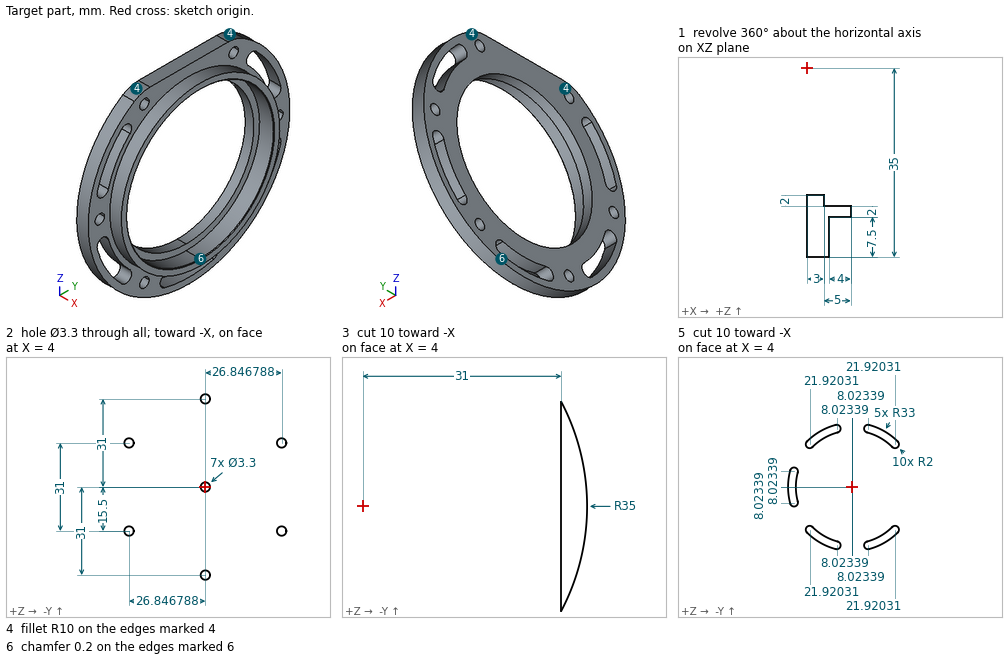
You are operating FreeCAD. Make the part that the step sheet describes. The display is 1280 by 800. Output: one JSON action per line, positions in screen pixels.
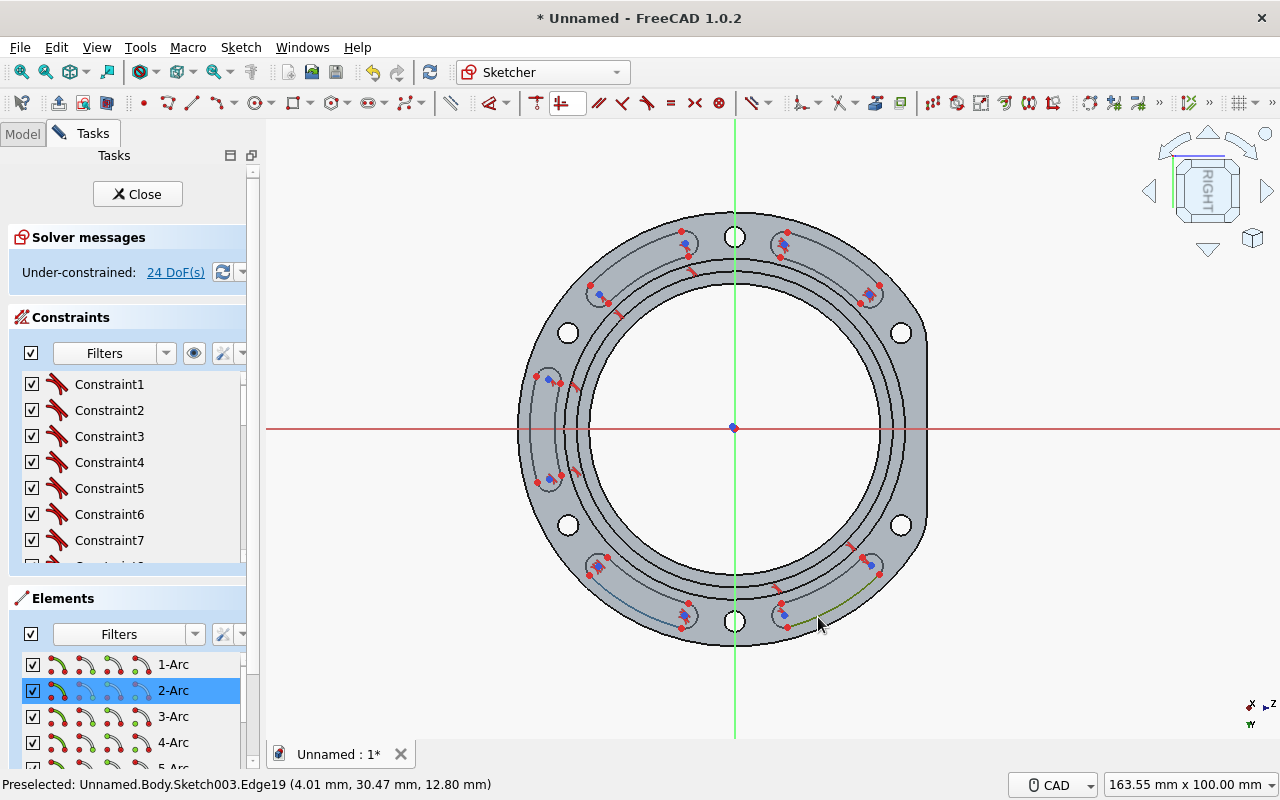
{"action": "left_click", "coordinate": [536, 104]}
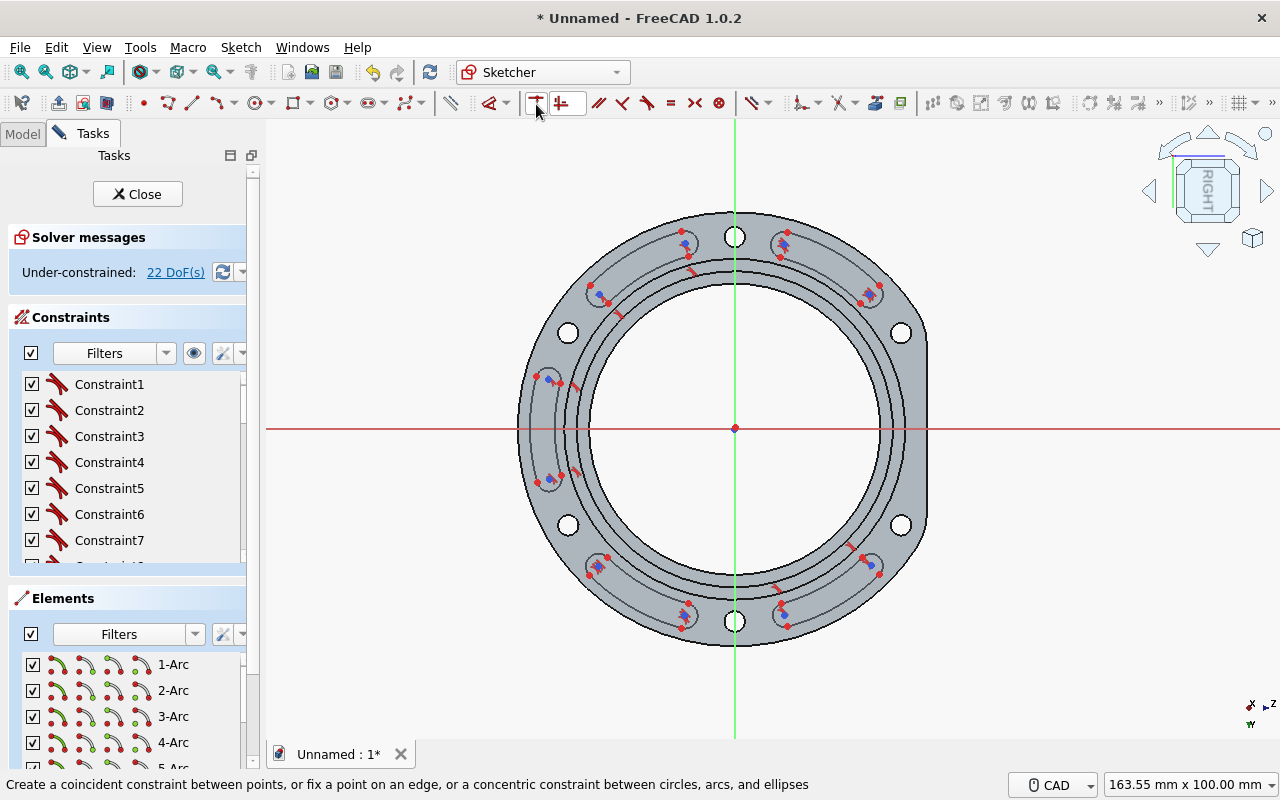
{"action": "scroll", "coordinate": [735, 429], "scroll_direction": "up", "scroll_amount": 7}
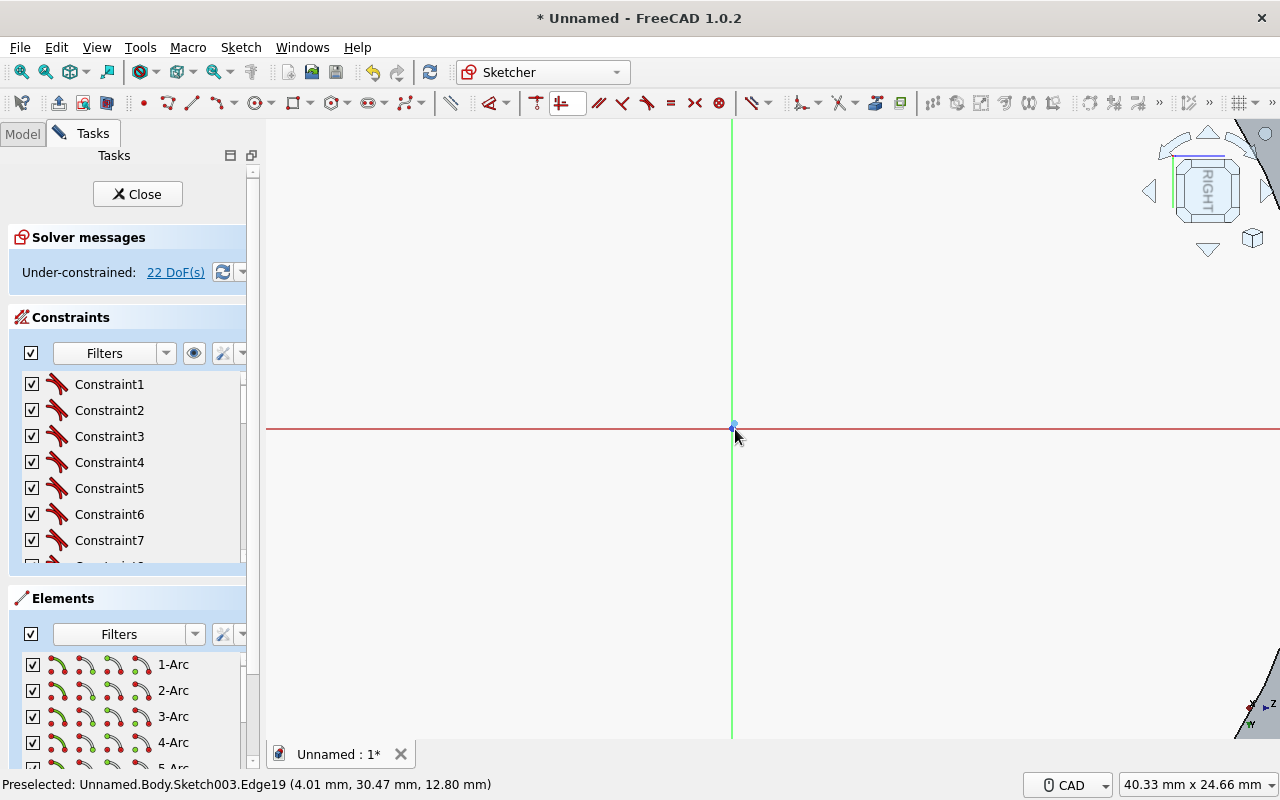
{"action": "left_click_drag", "start_coordinate": [723, 413], "coordinate": [745, 439]}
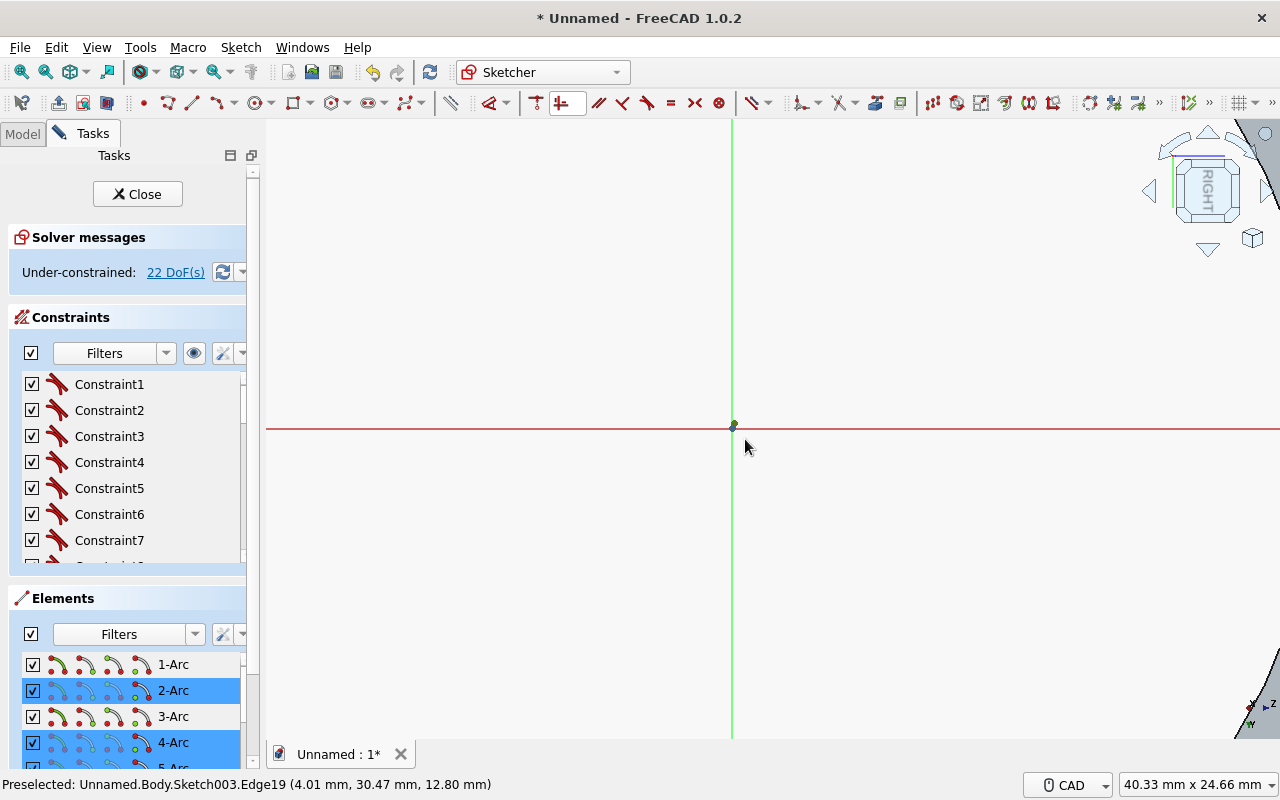
{"action": "left_click", "coordinate": [536, 104]}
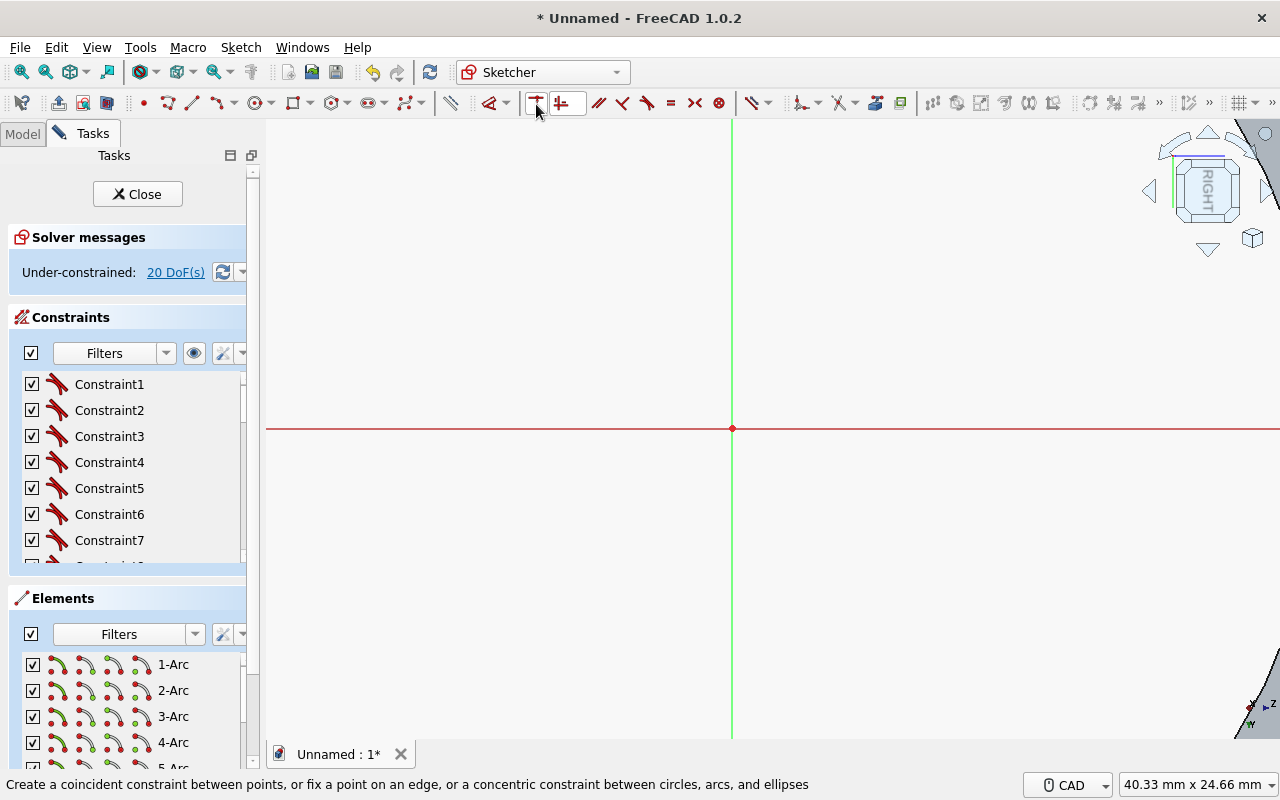
{"action": "scroll", "coordinate": [735, 429], "scroll_direction": "down", "scroll_amount": 7}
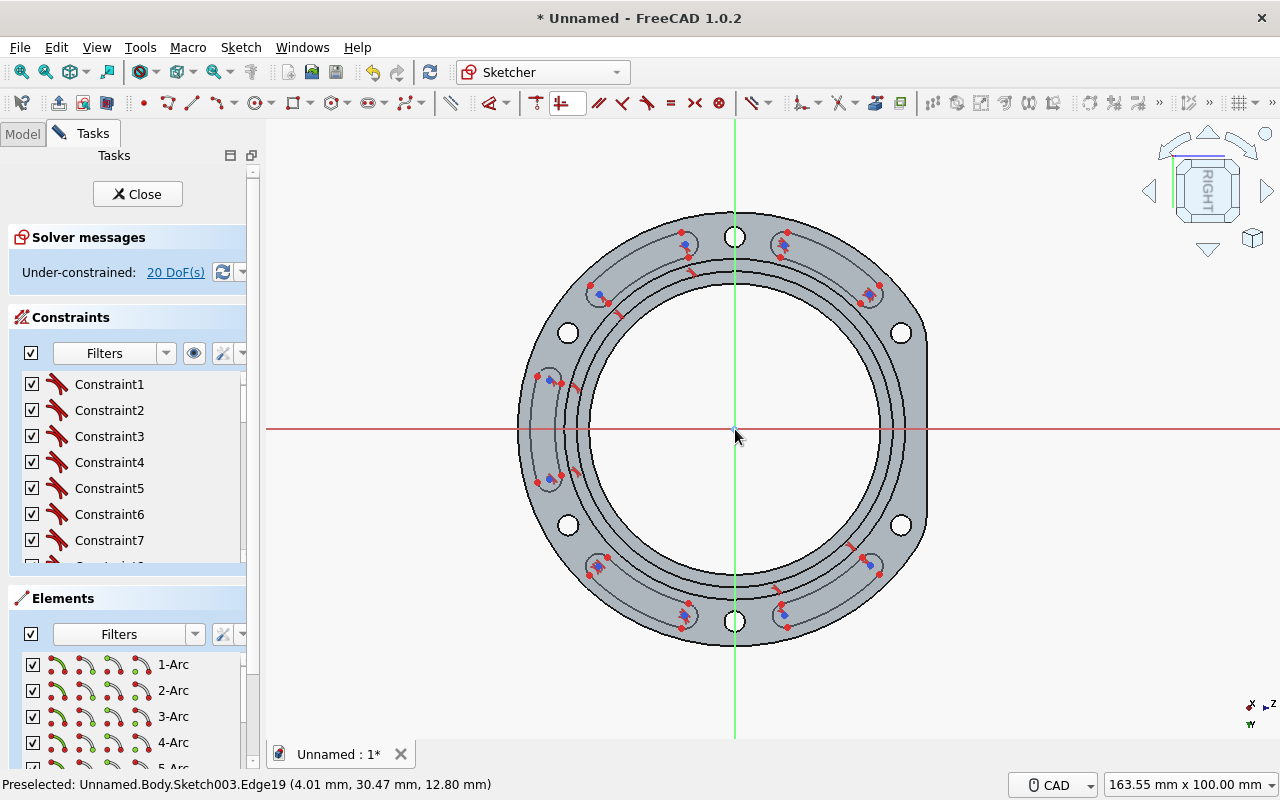
{"action": "left_click", "coordinate": [629, 576]}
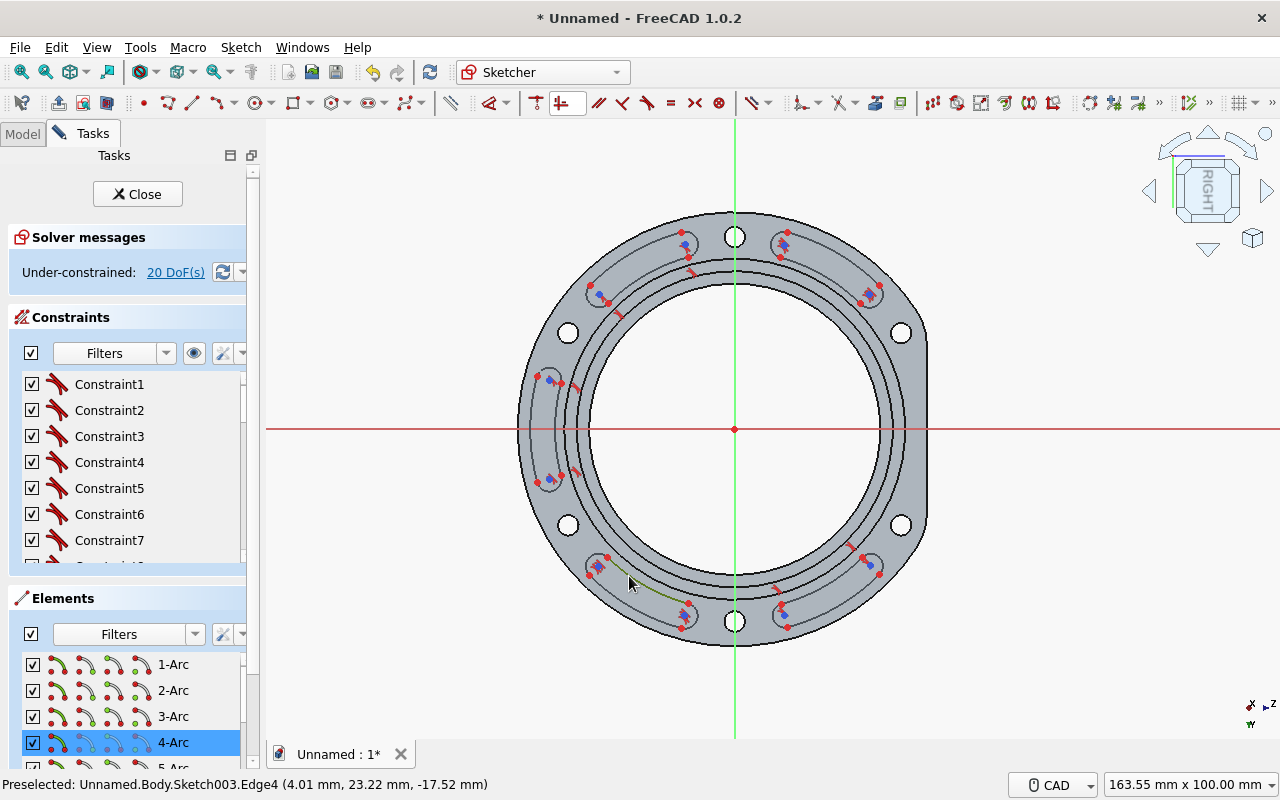
{"action": "left_click", "coordinate": [556, 411]}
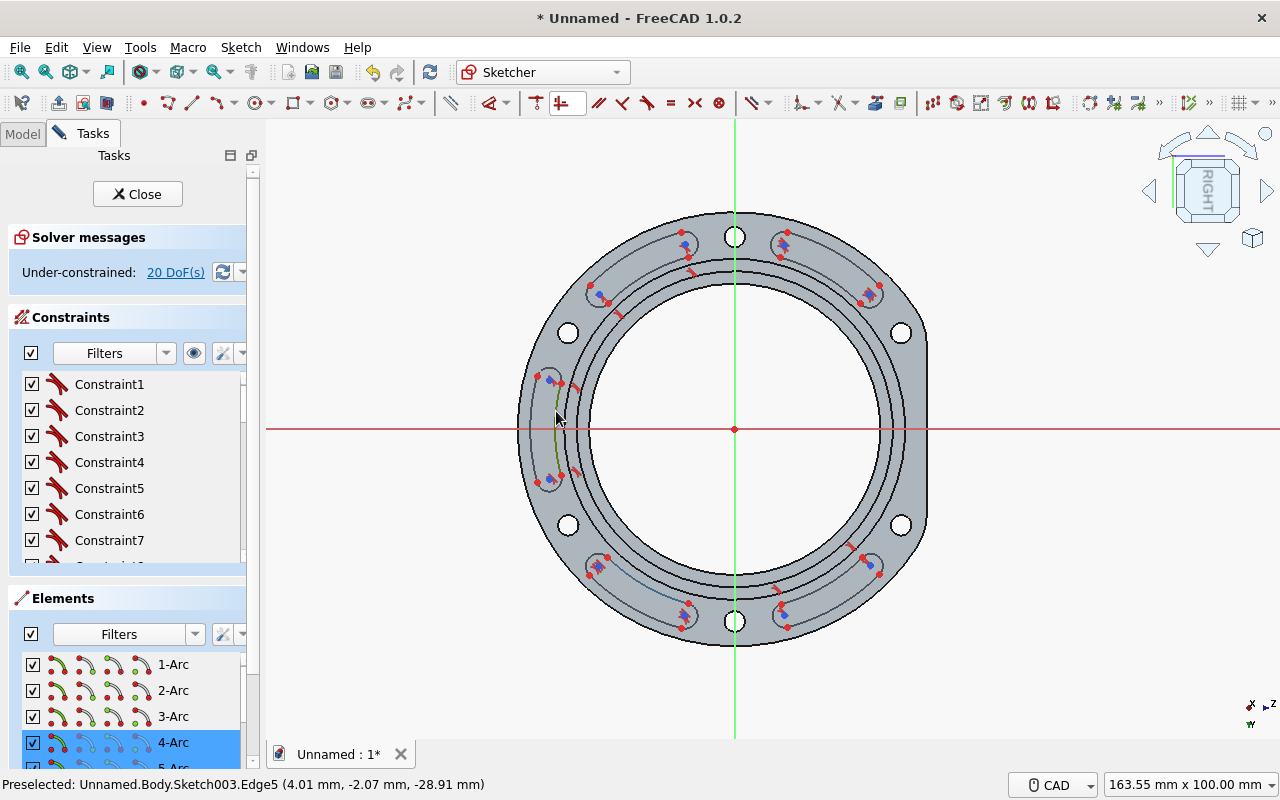
{"action": "left_click", "coordinate": [662, 267]}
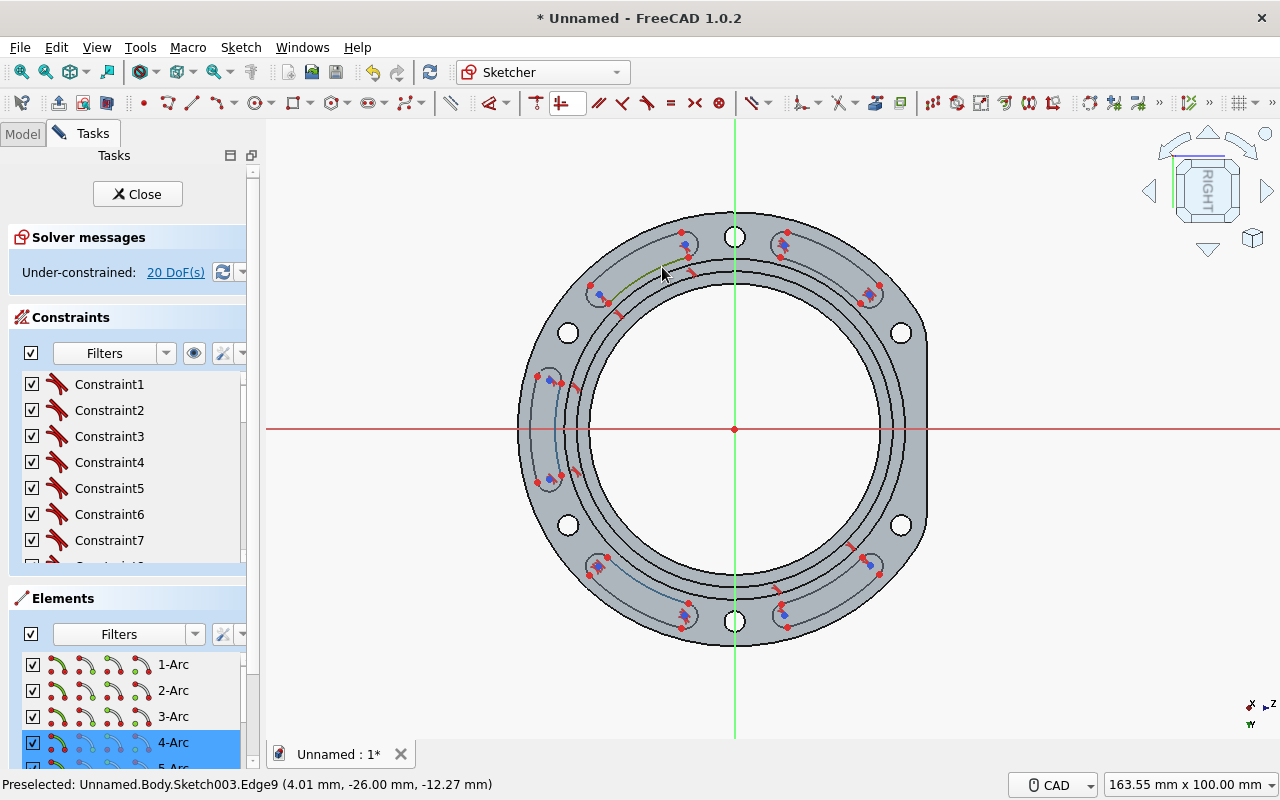
{"action": "left_click", "coordinate": [839, 286]}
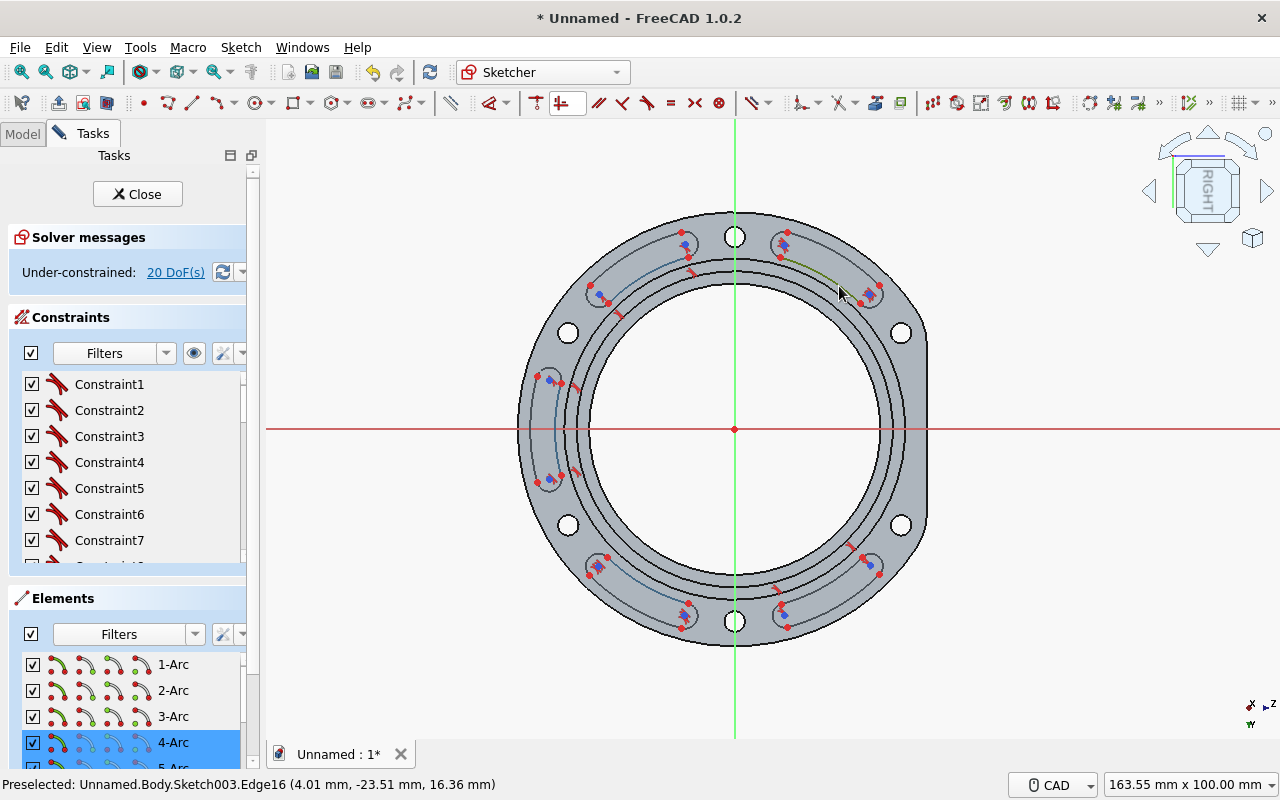
{"action": "left_click", "coordinate": [808, 595]}